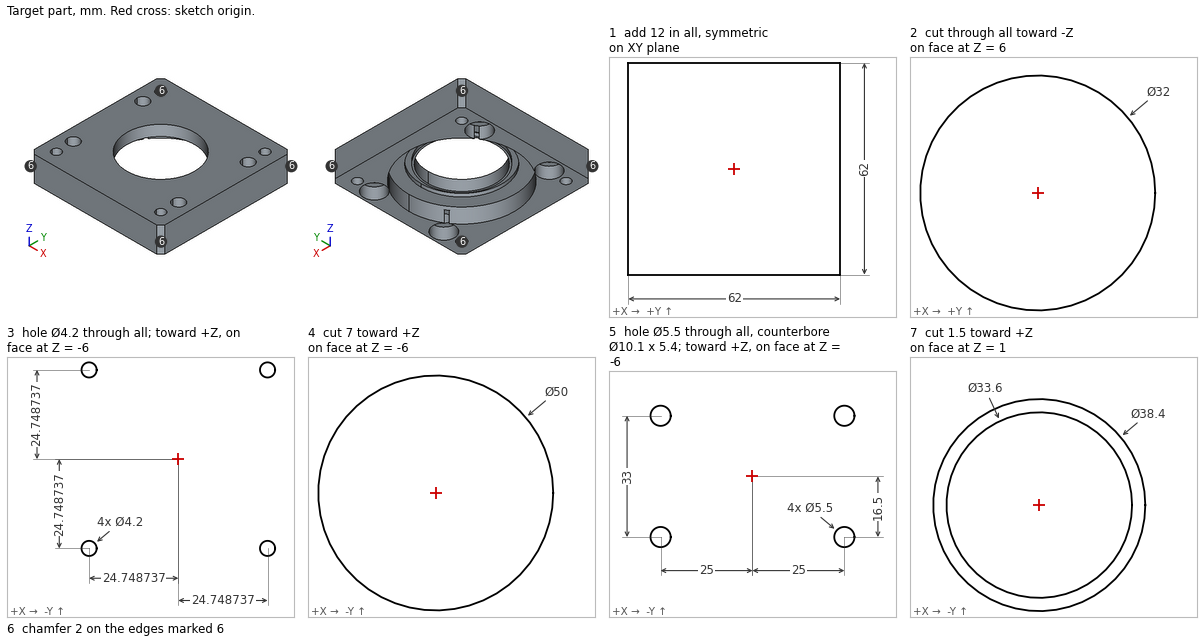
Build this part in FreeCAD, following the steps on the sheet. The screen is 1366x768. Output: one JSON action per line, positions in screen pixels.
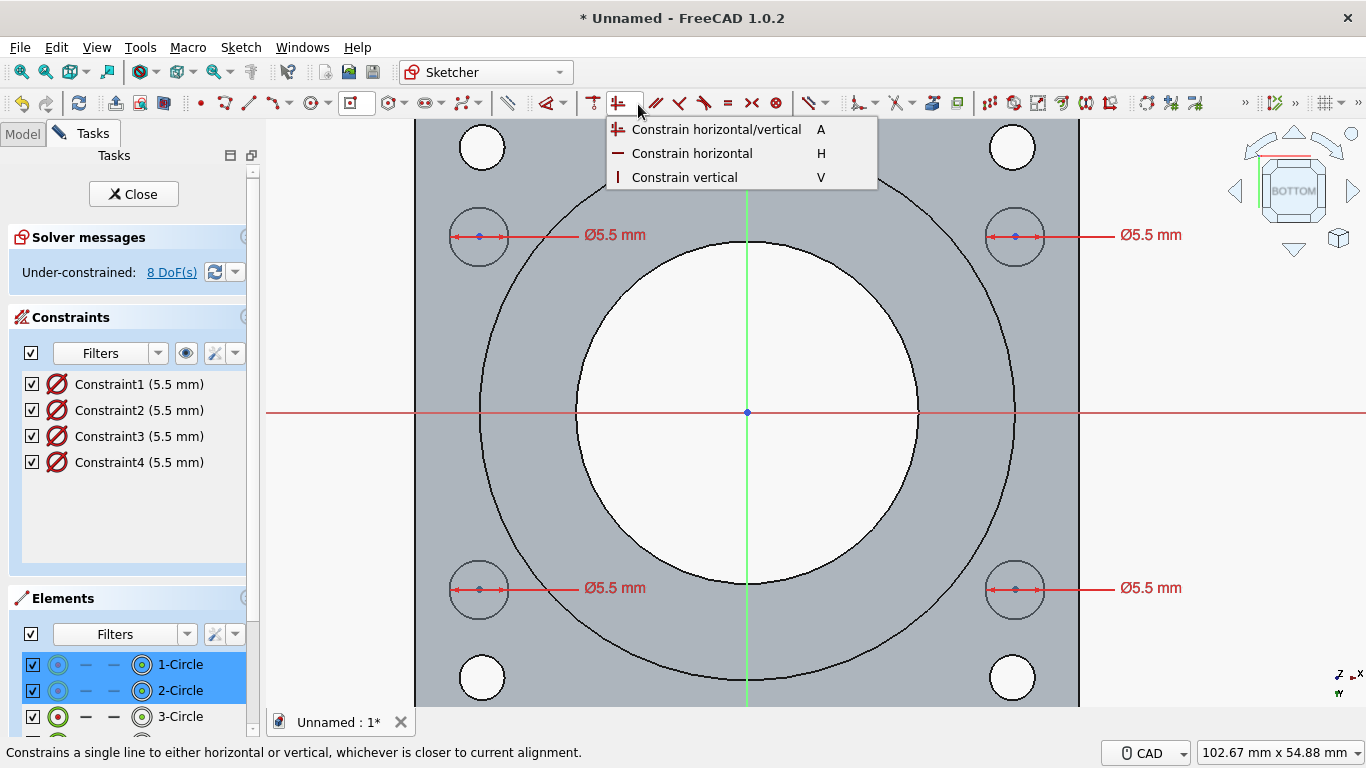
{"action": "left_click", "coordinate": [742, 153]}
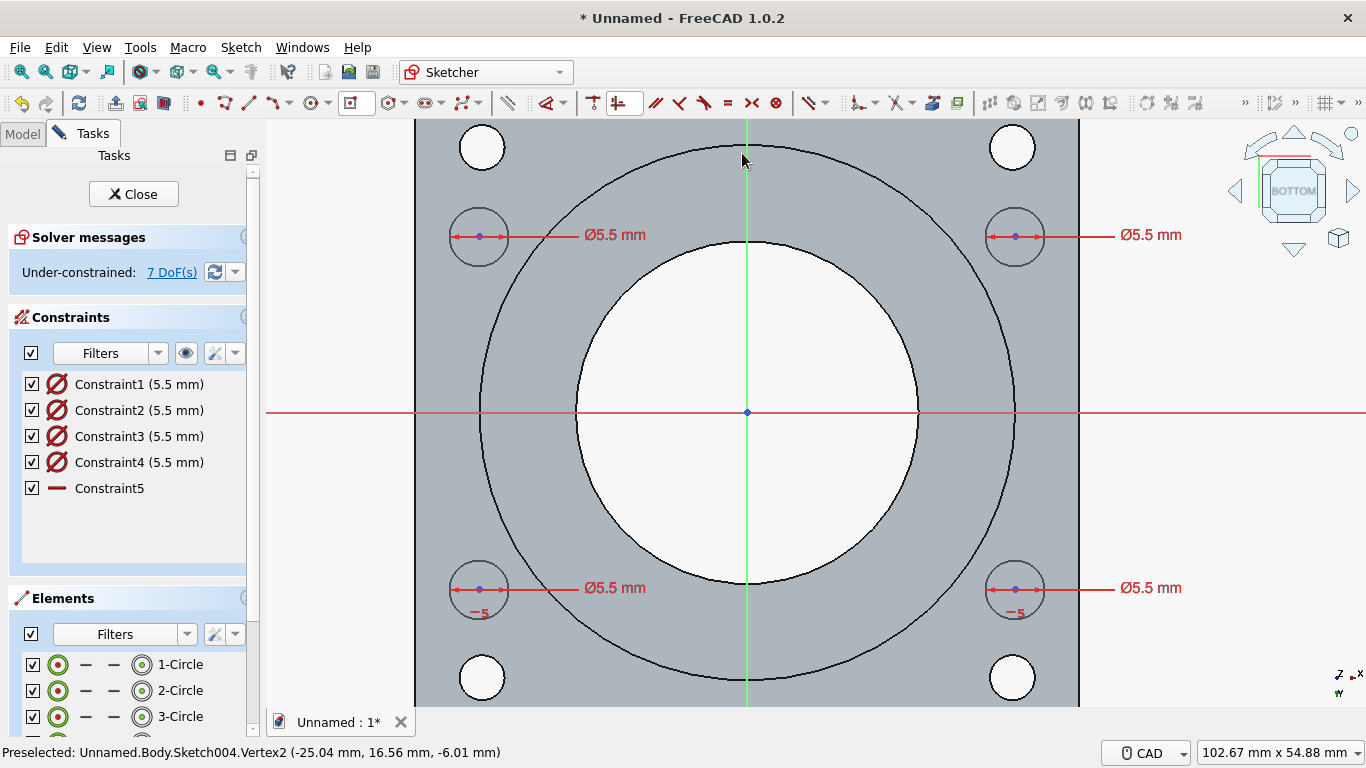
{"action": "left_click", "coordinate": [479, 590]}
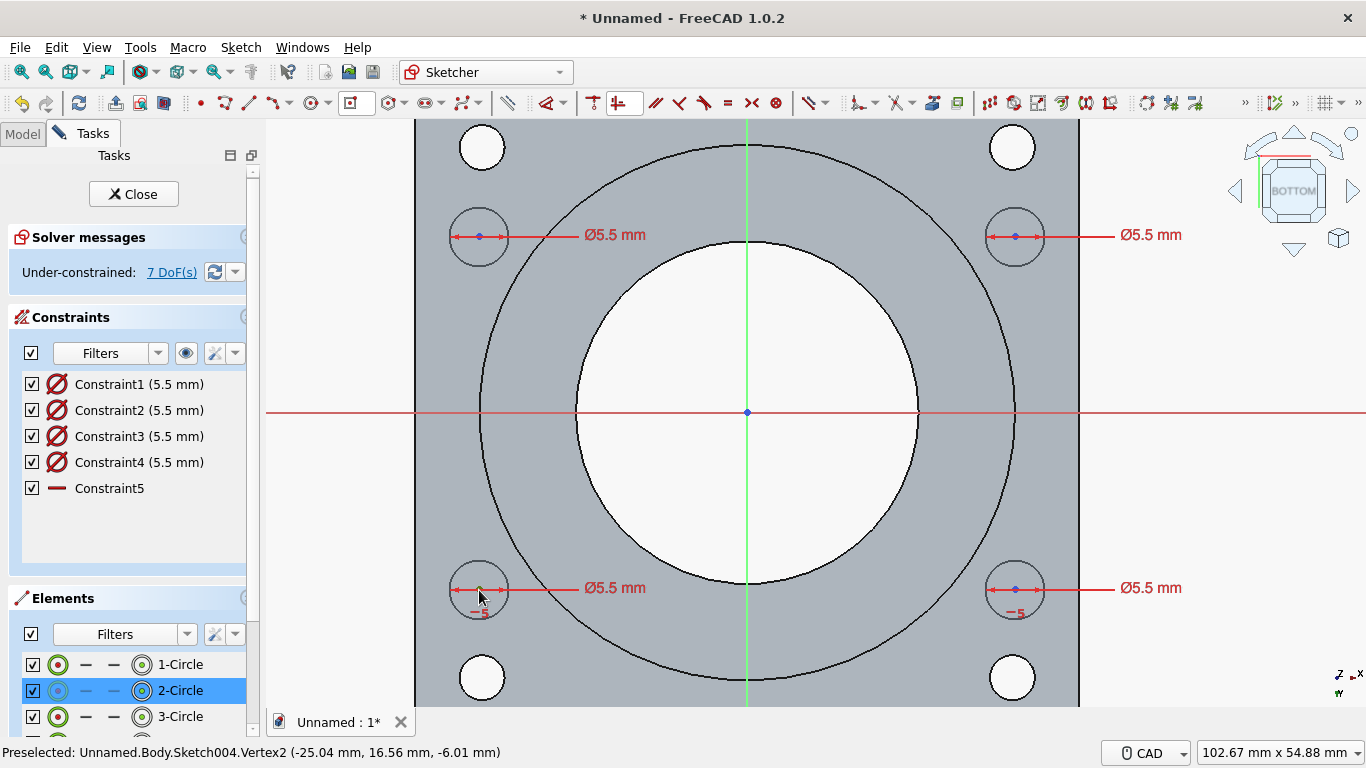
{"action": "left_click", "coordinate": [479, 237]}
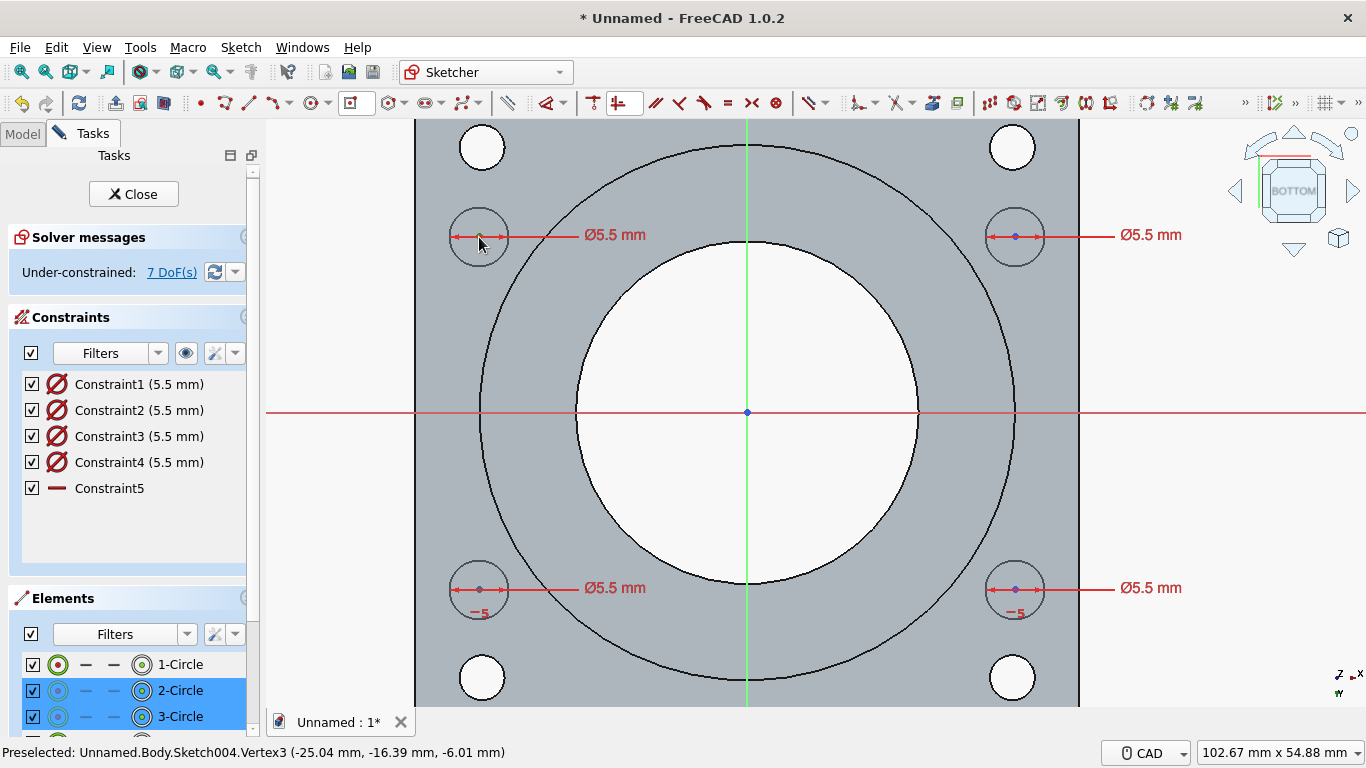
{"action": "key", "text": "v"}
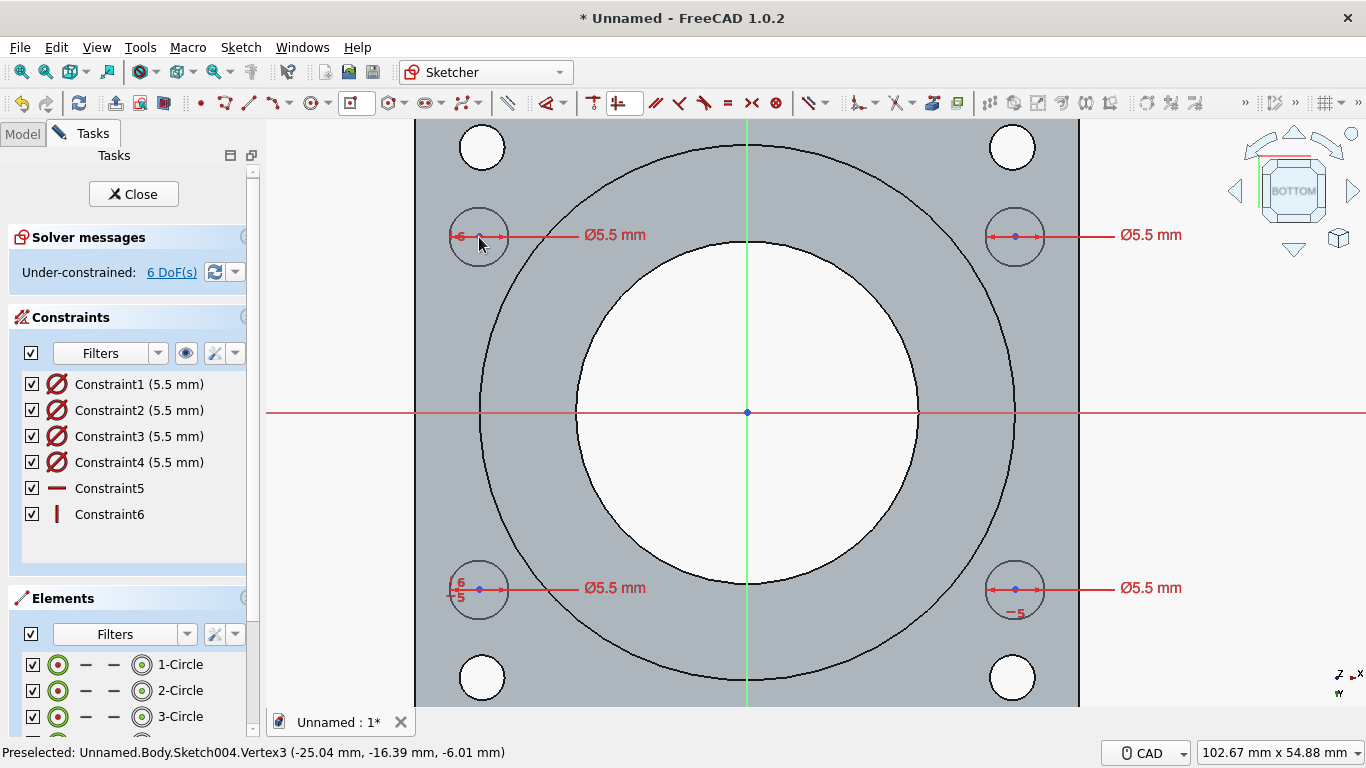
{"action": "left_click", "coordinate": [1015, 590]}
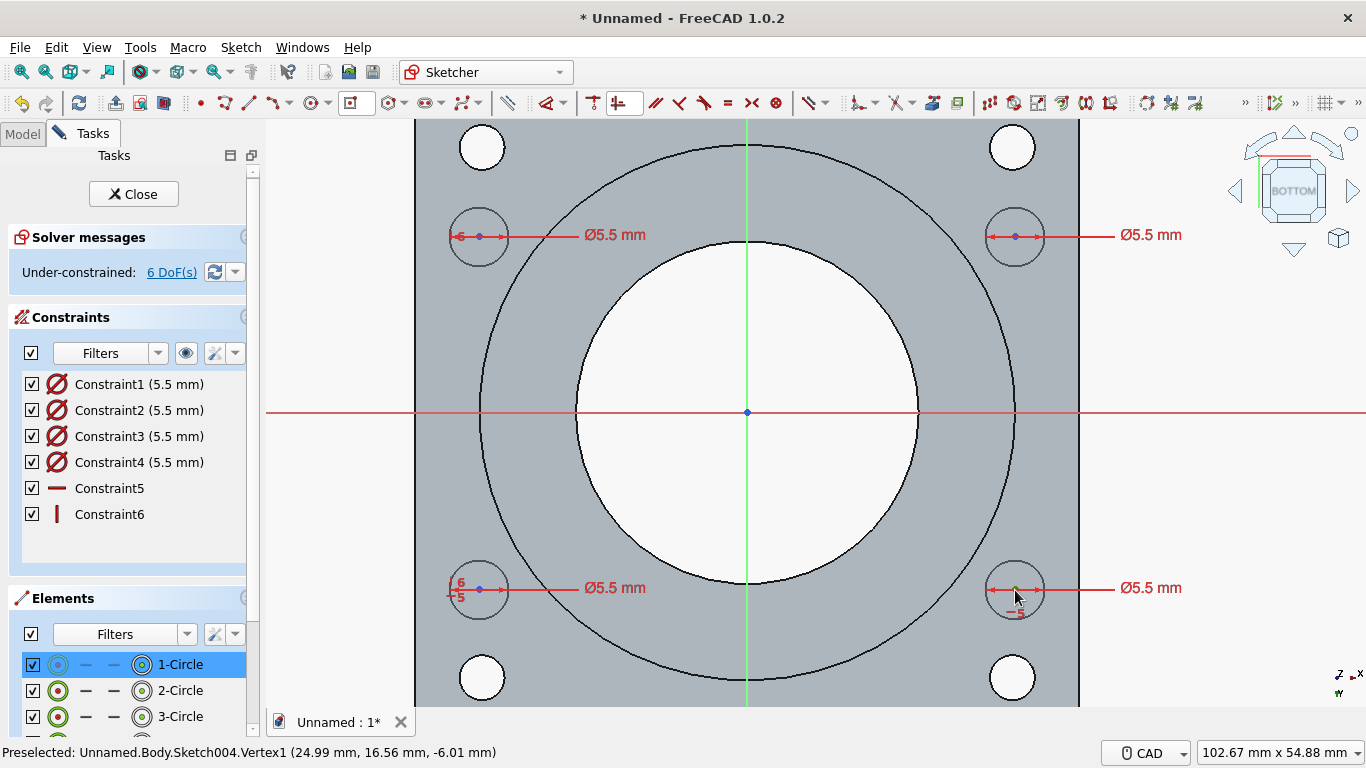
{"action": "left_click", "coordinate": [1015, 237]}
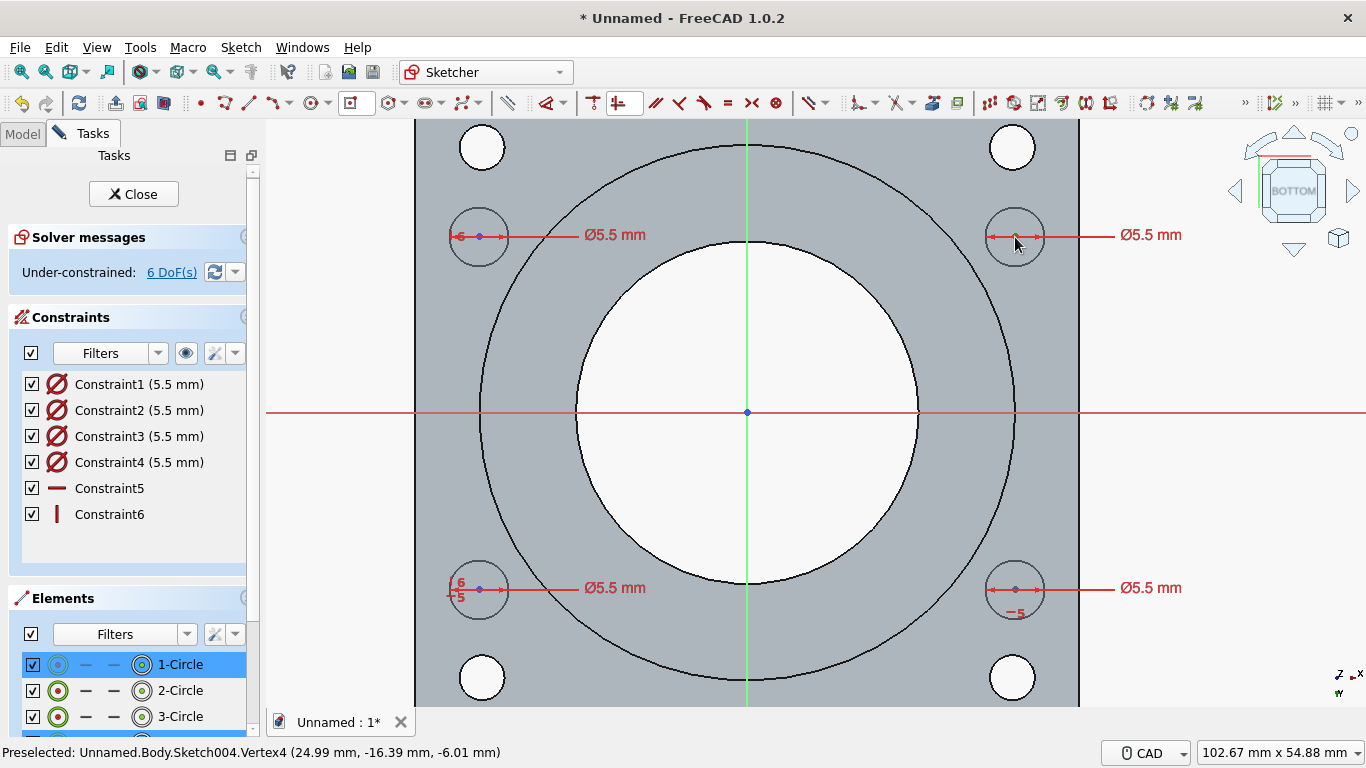
{"action": "left_click", "coordinate": [638, 104]}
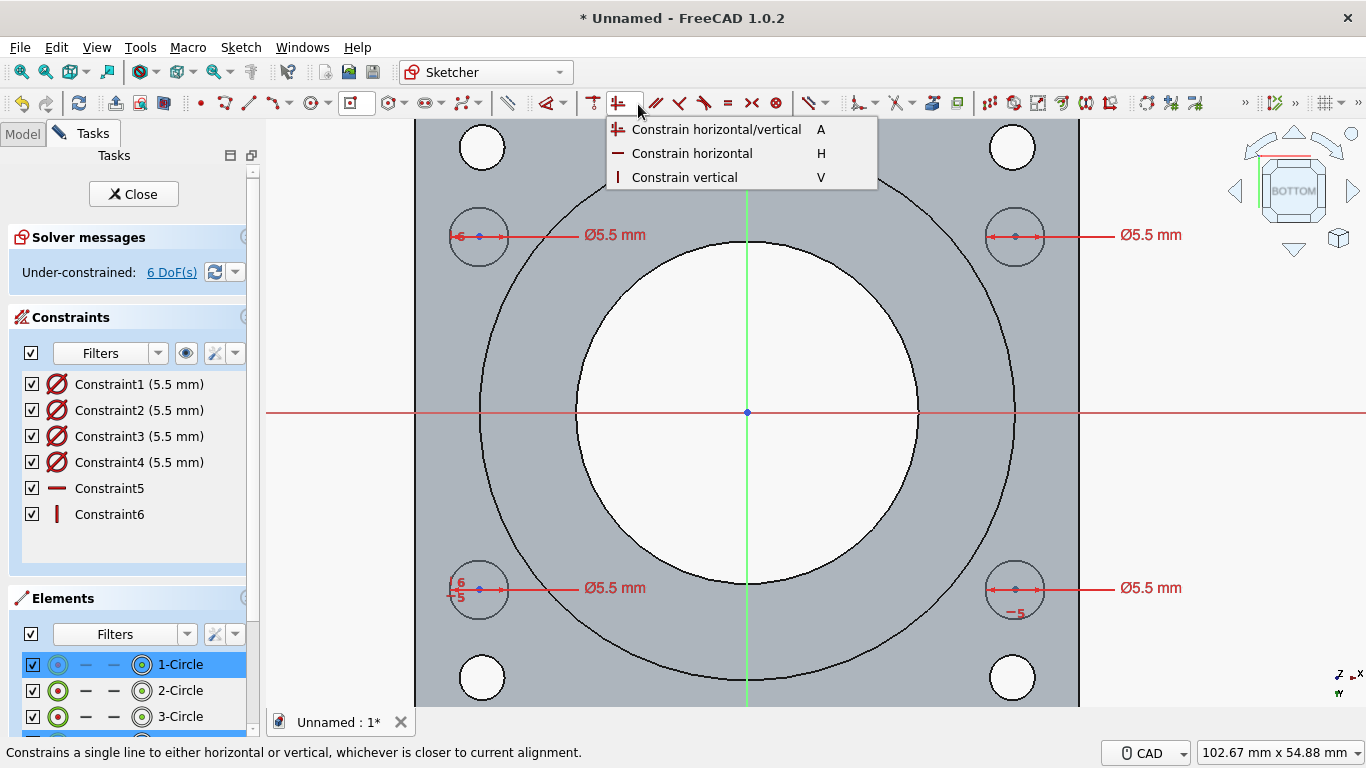
{"action": "left_click", "coordinate": [742, 177]}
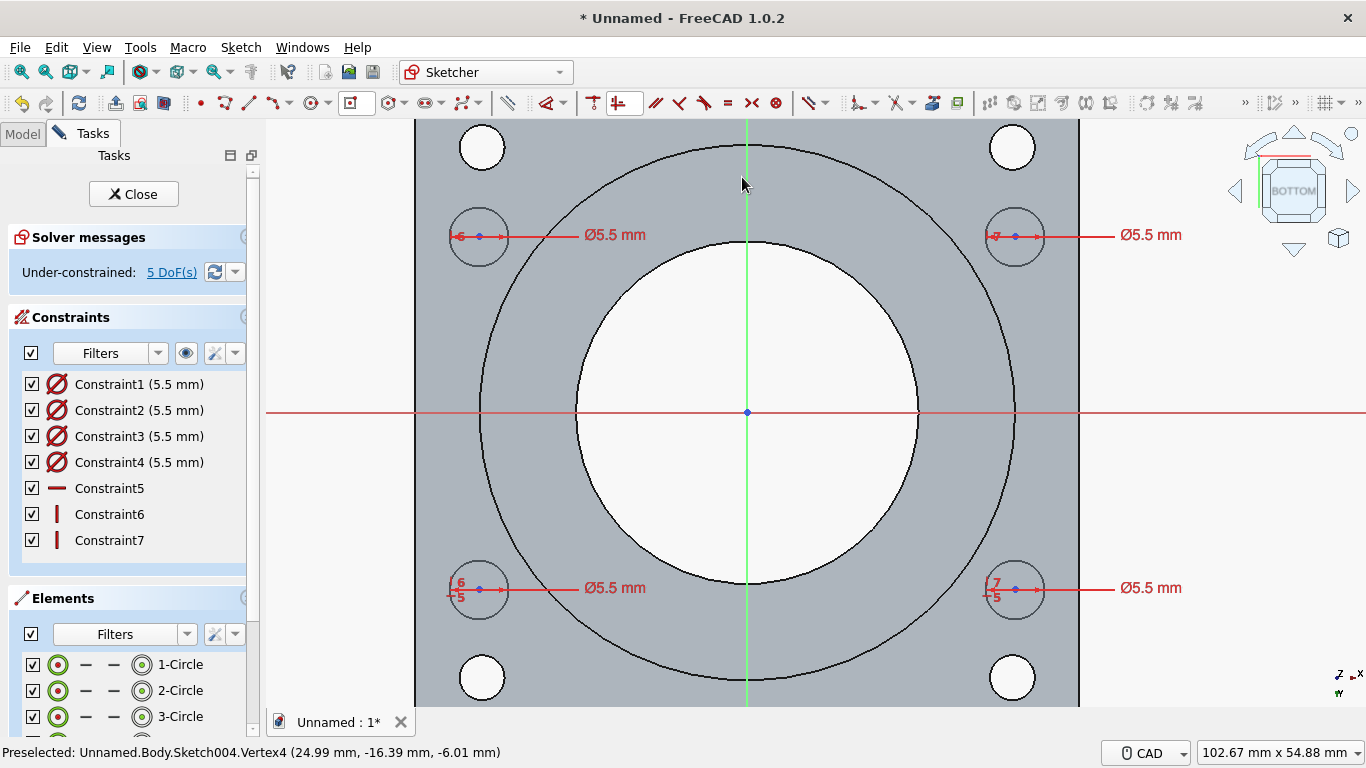
{"action": "left_click", "coordinate": [479, 237]}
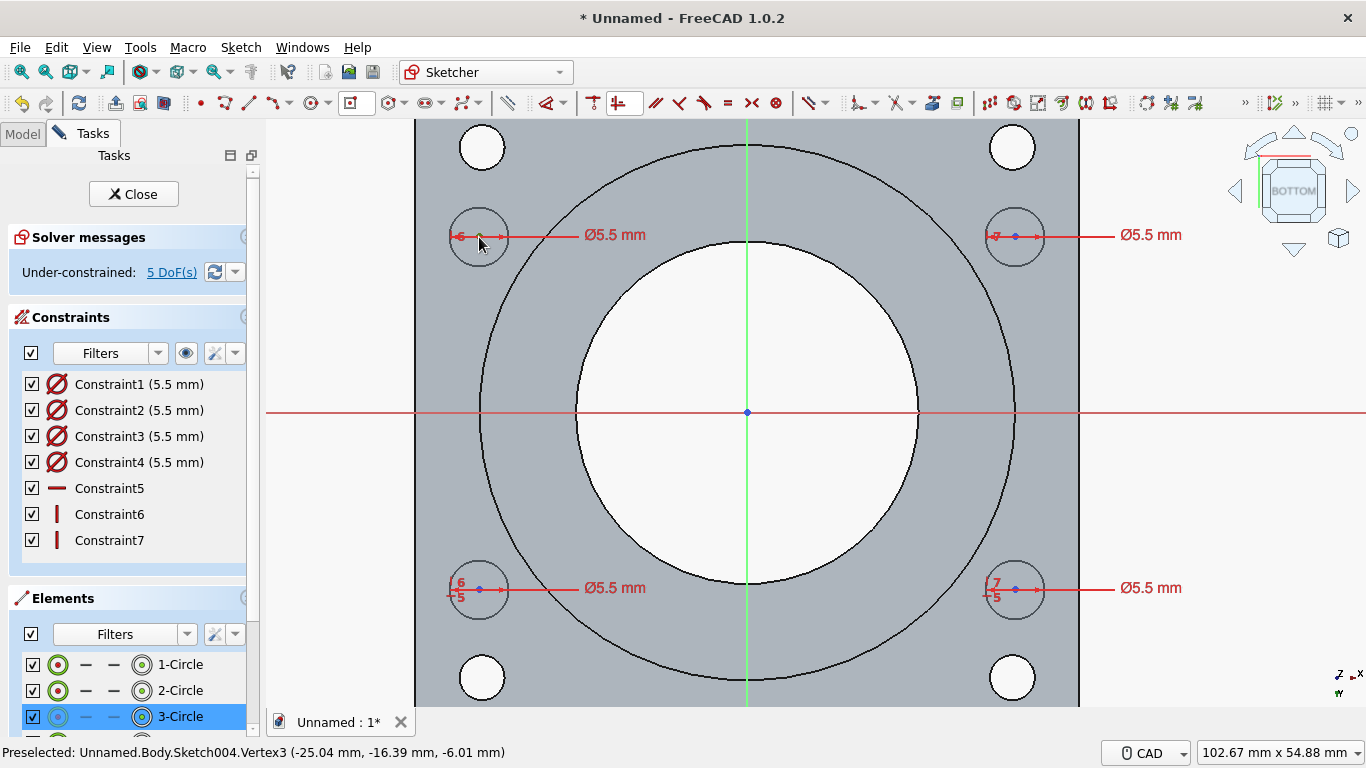
{"action": "left_click", "coordinate": [1015, 237]}